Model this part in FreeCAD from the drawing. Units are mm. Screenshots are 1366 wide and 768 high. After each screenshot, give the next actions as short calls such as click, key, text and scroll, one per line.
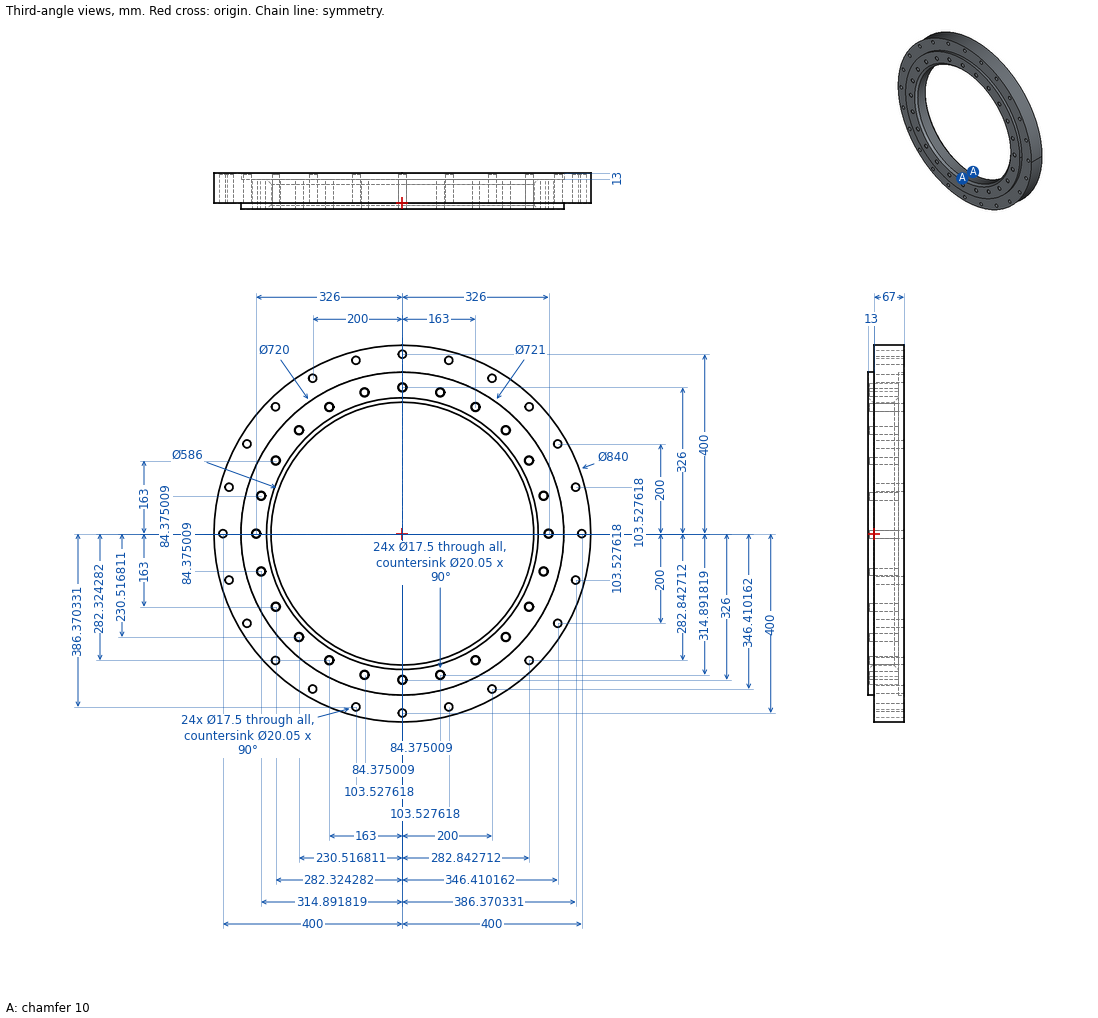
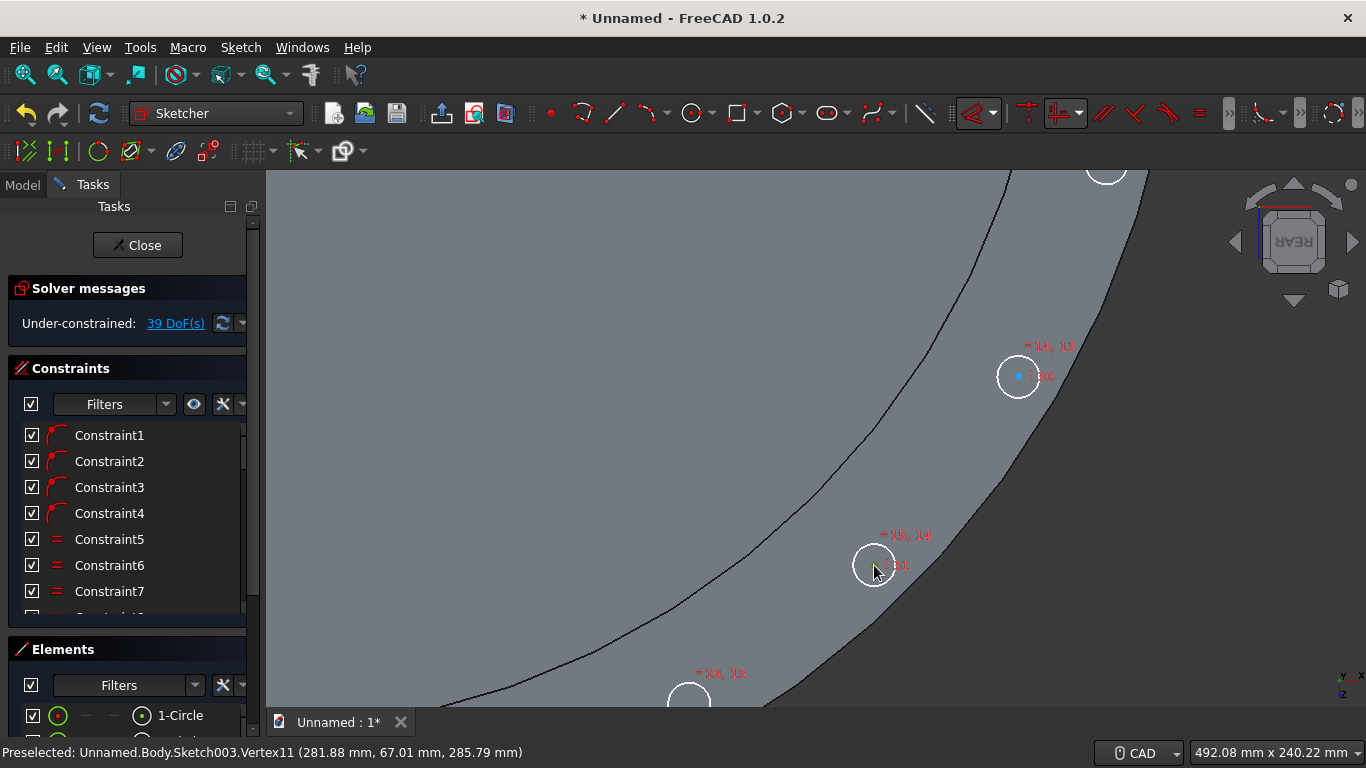
scroll(875, 568, down, 8)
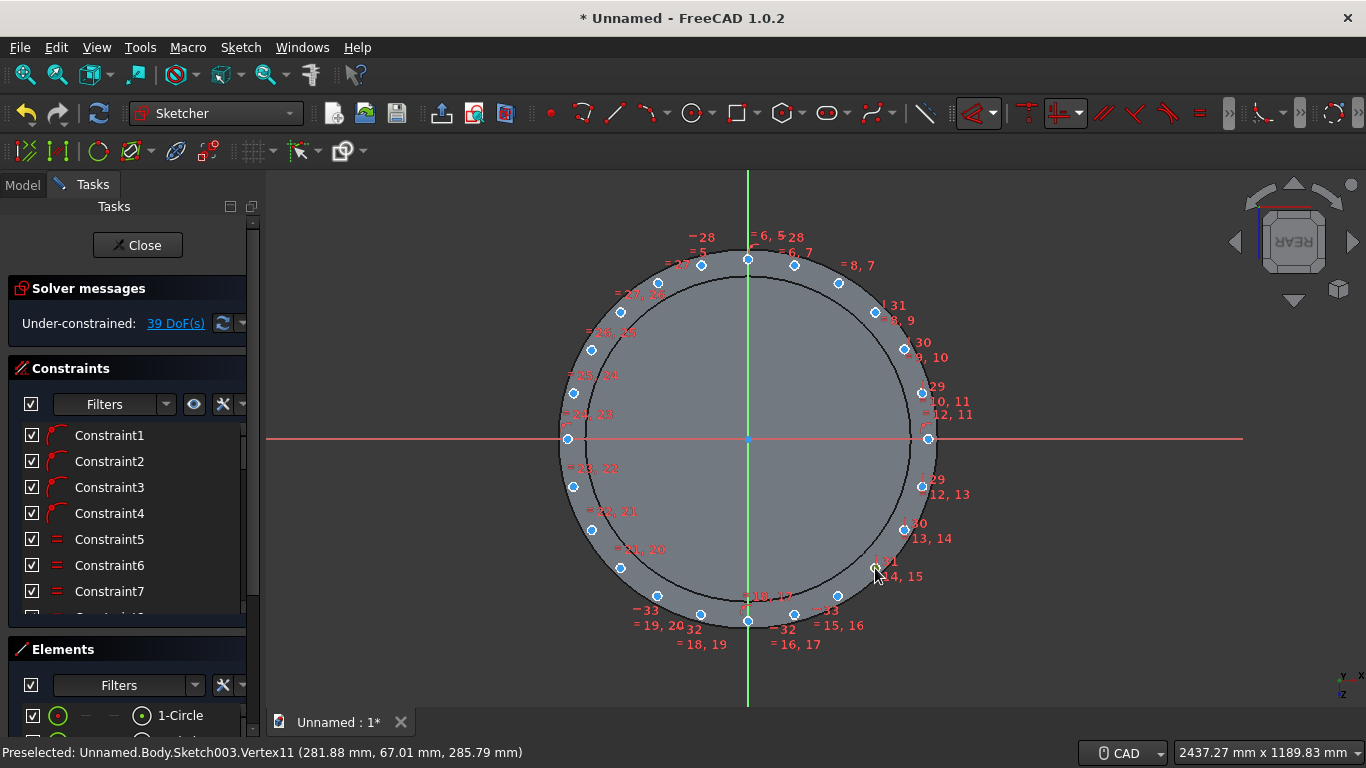
click(621, 568)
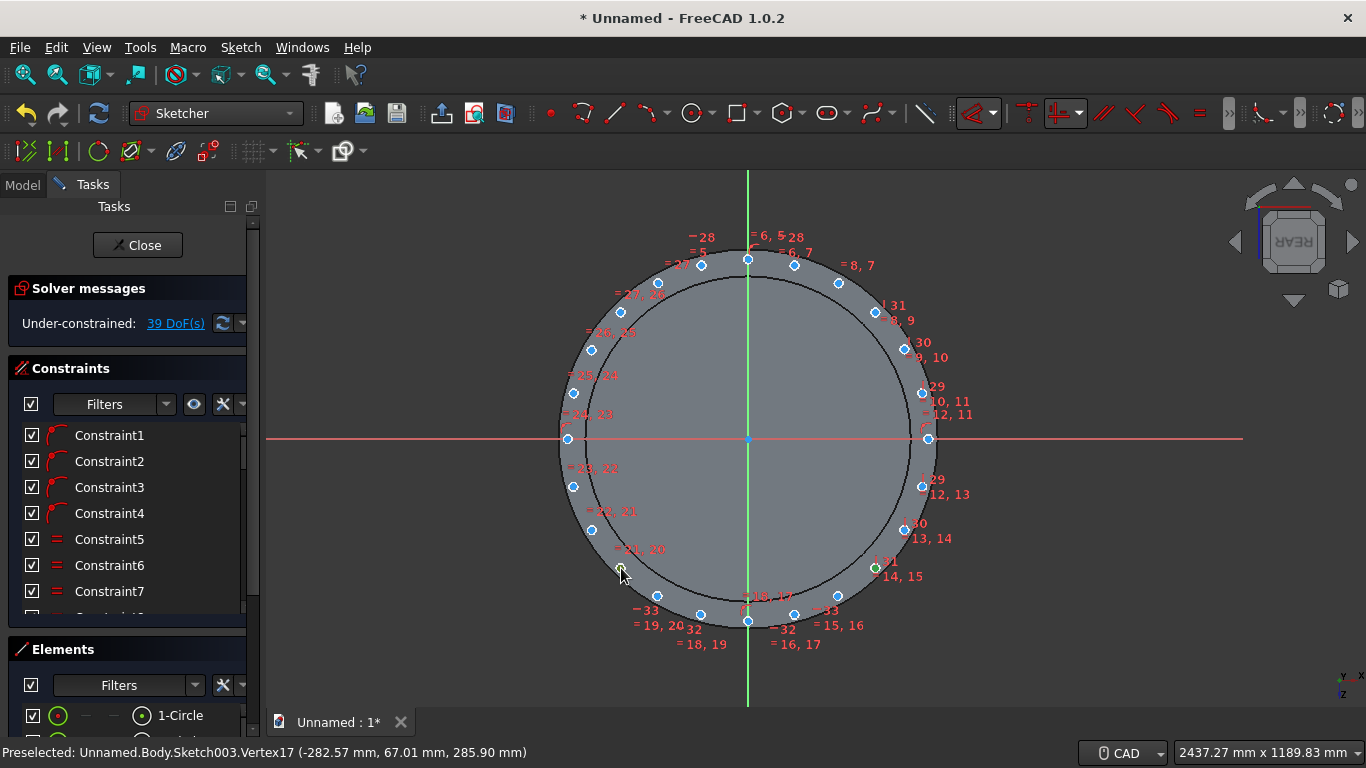
key(h)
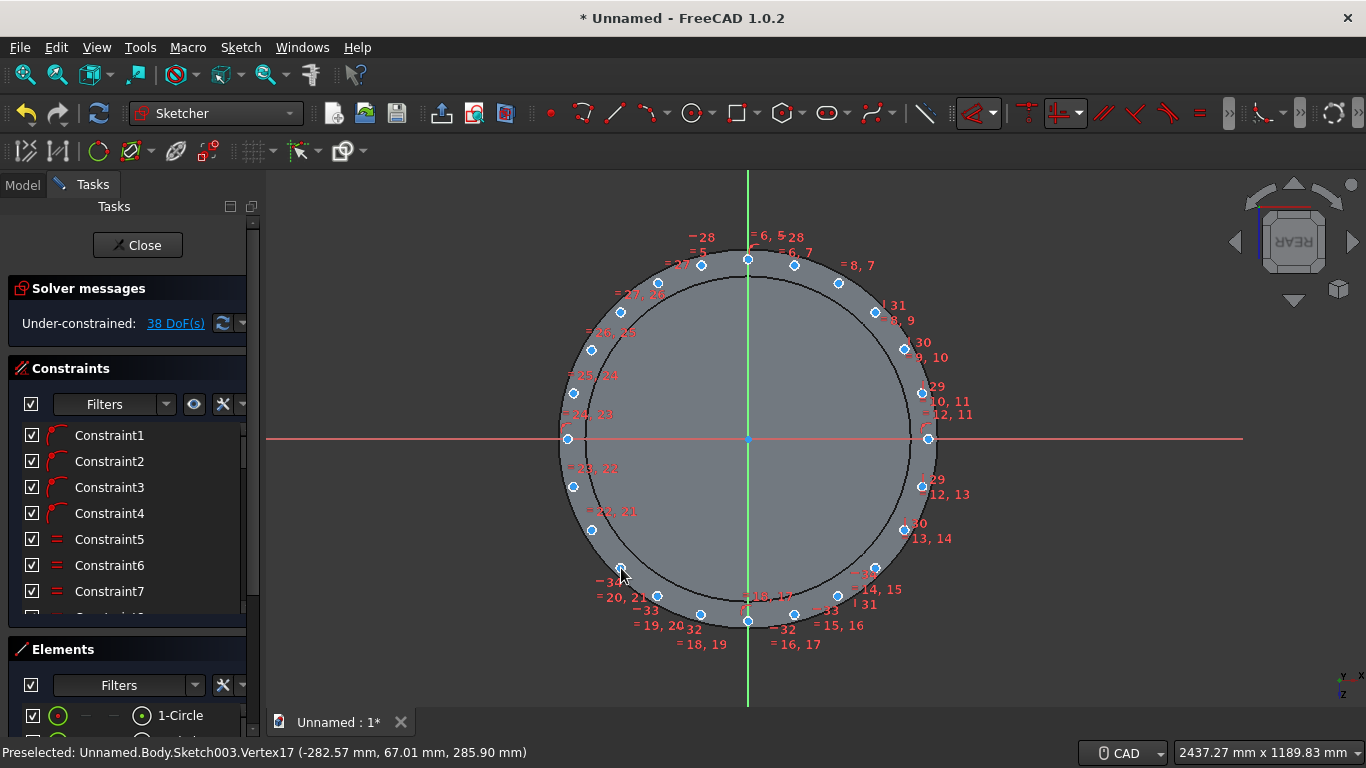
click(573, 487)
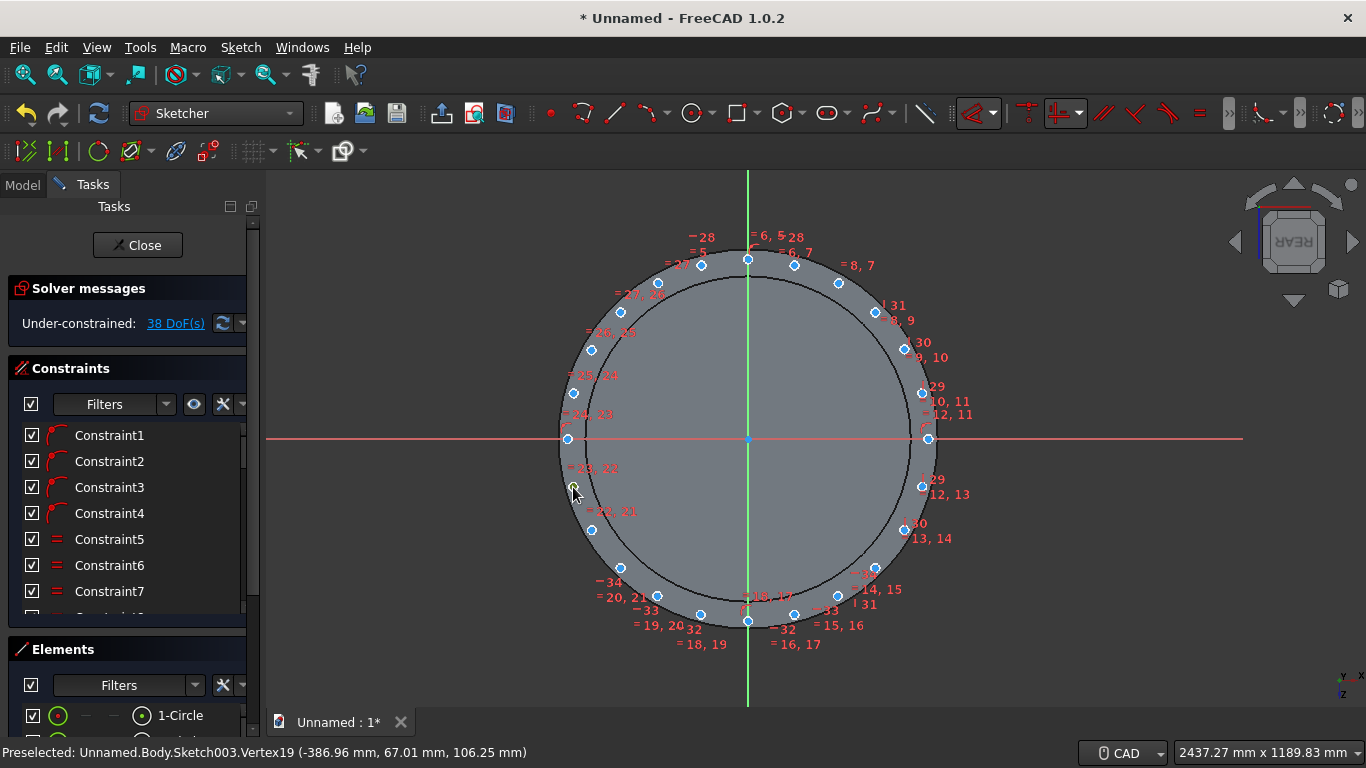
click(574, 393)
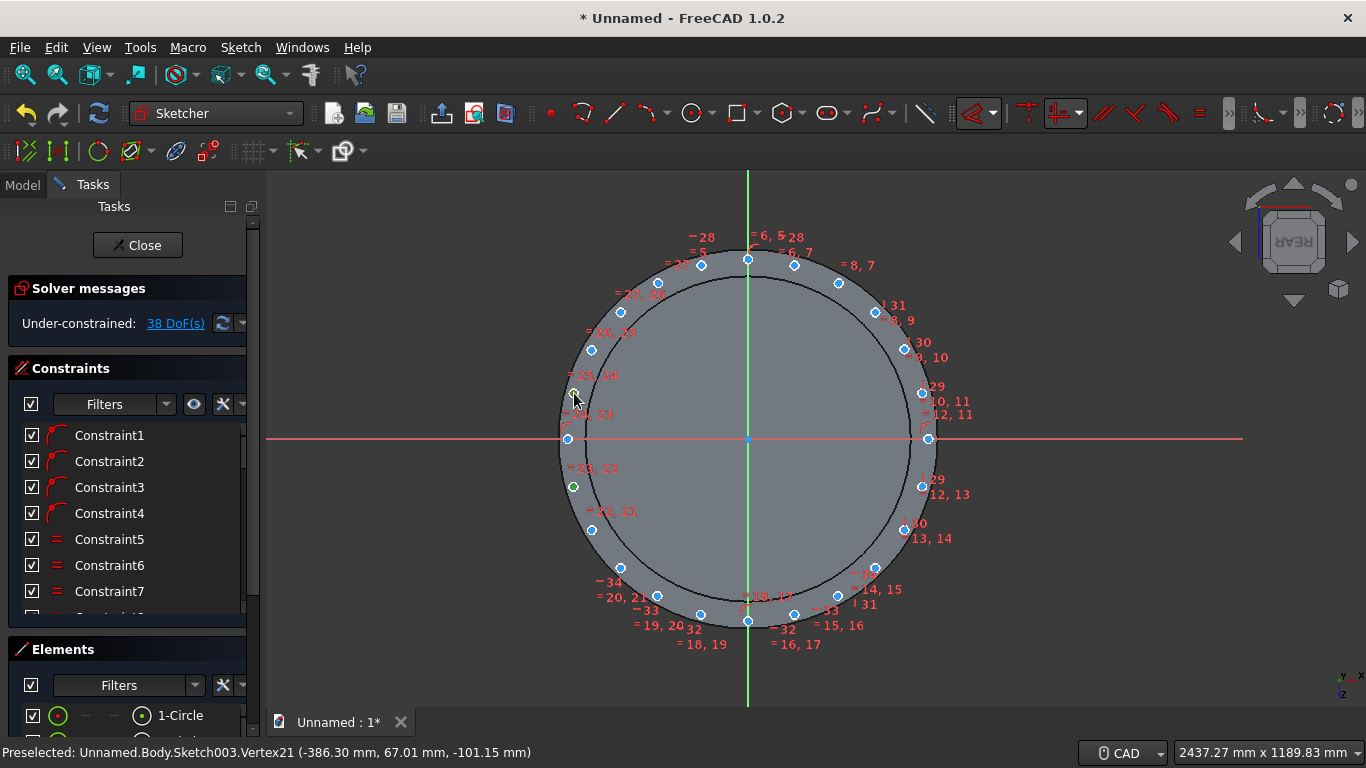
key(v)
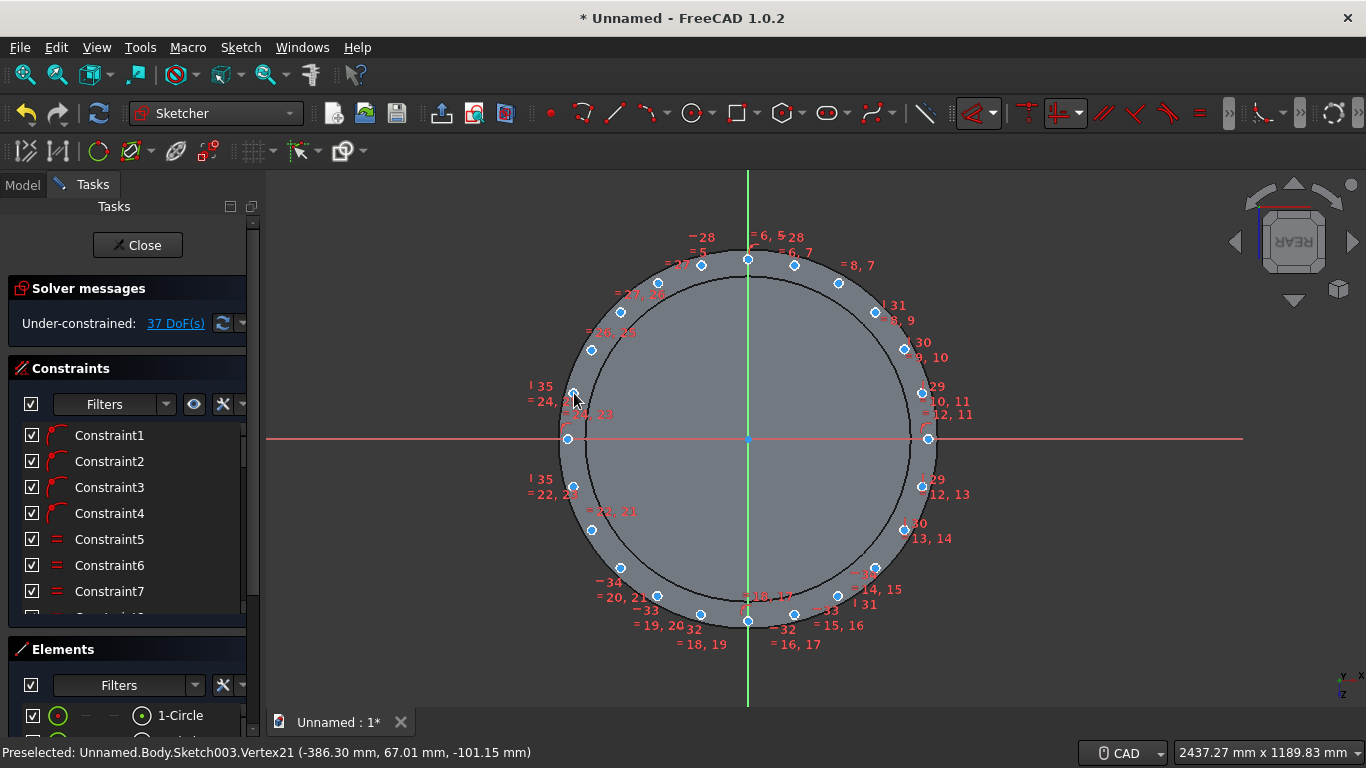
click(592, 530)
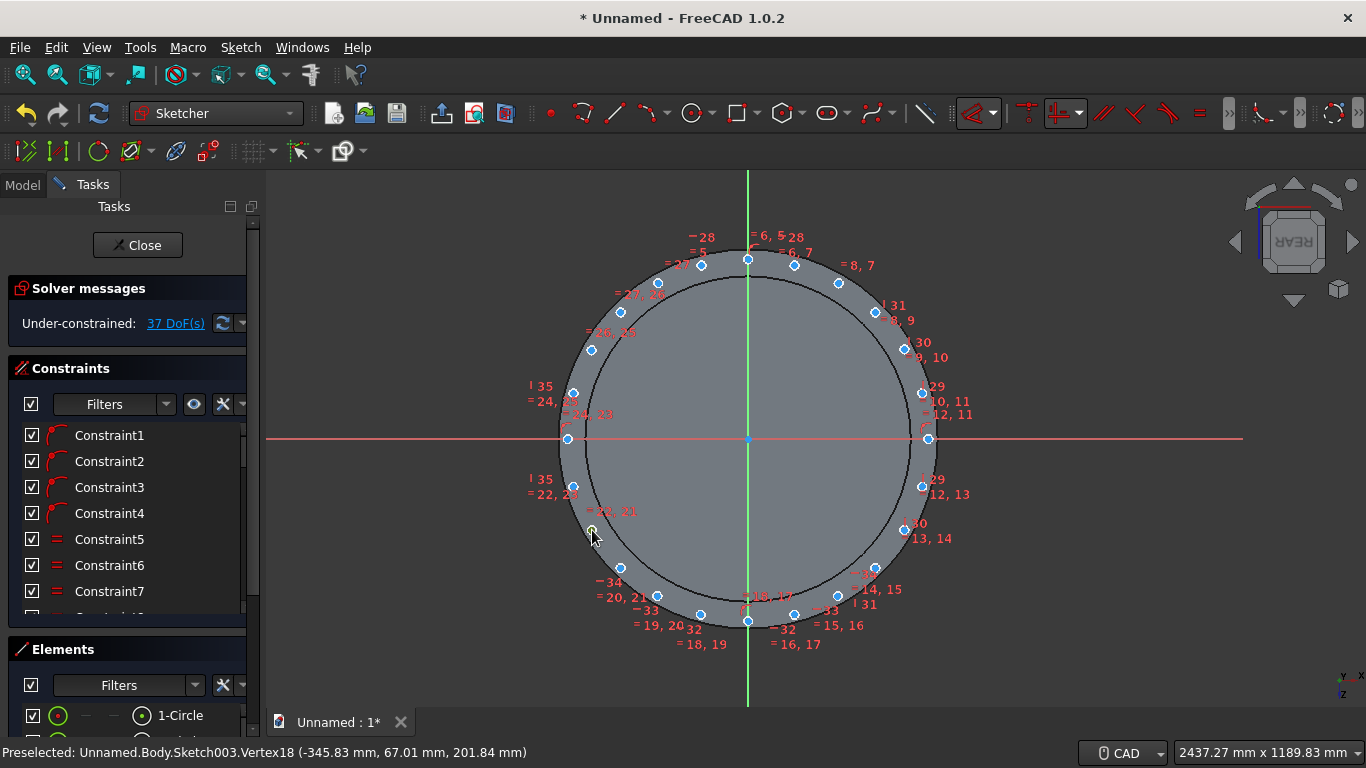
click(592, 350)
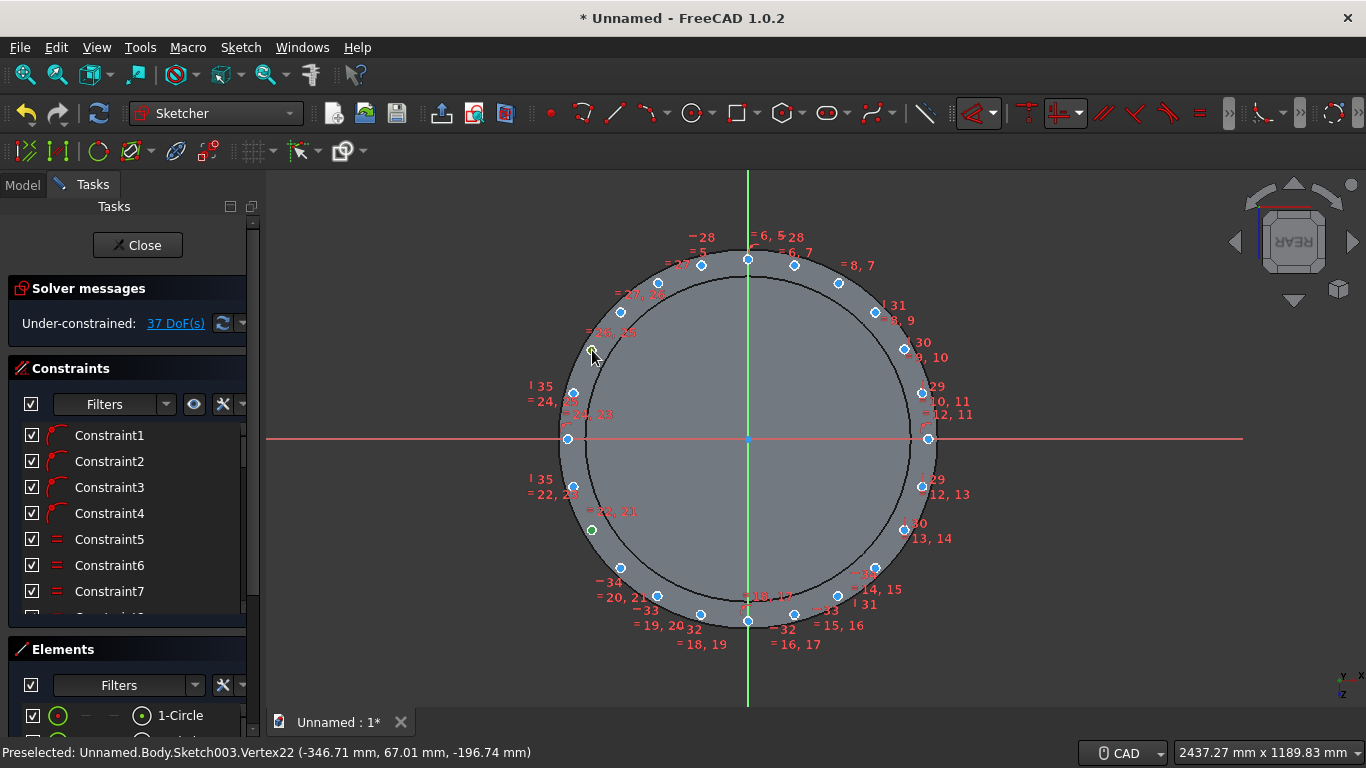
key(v)